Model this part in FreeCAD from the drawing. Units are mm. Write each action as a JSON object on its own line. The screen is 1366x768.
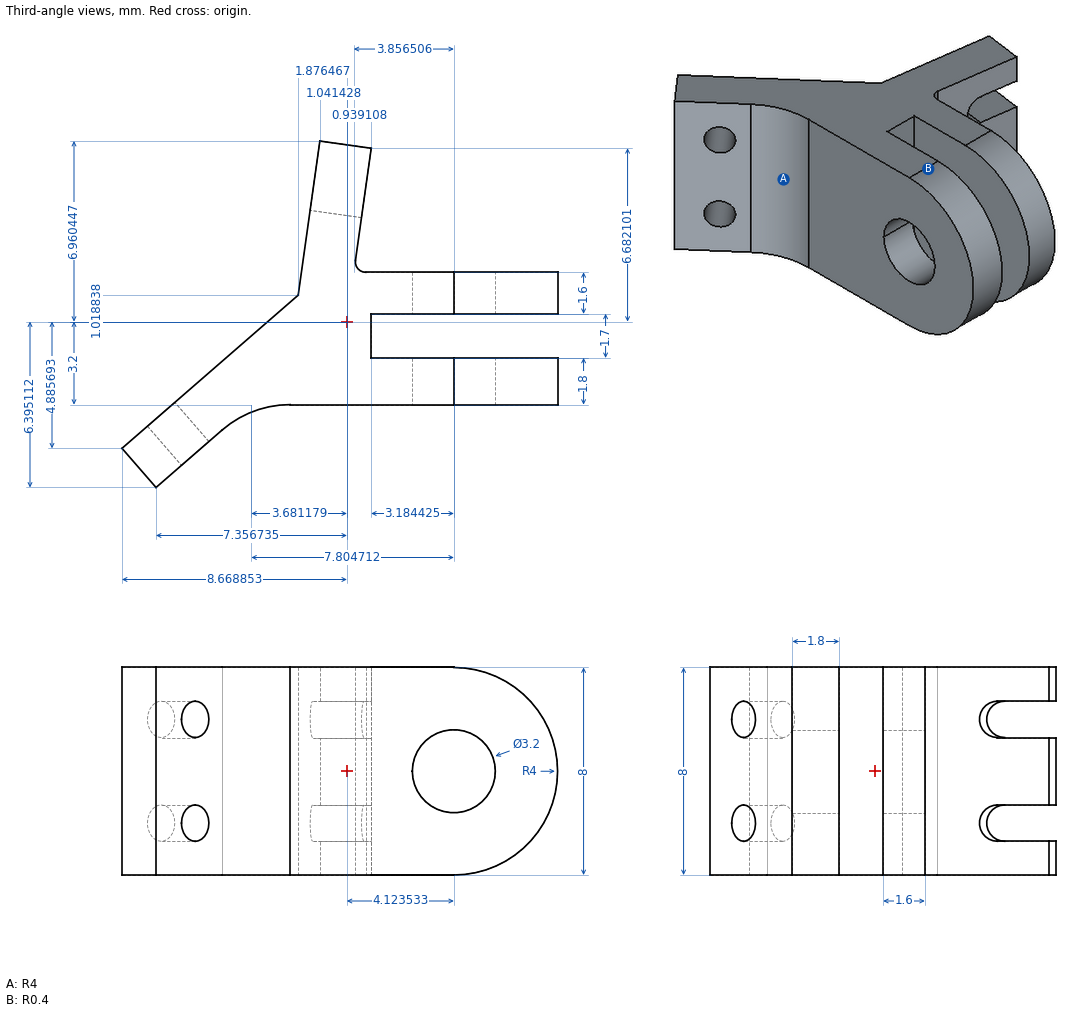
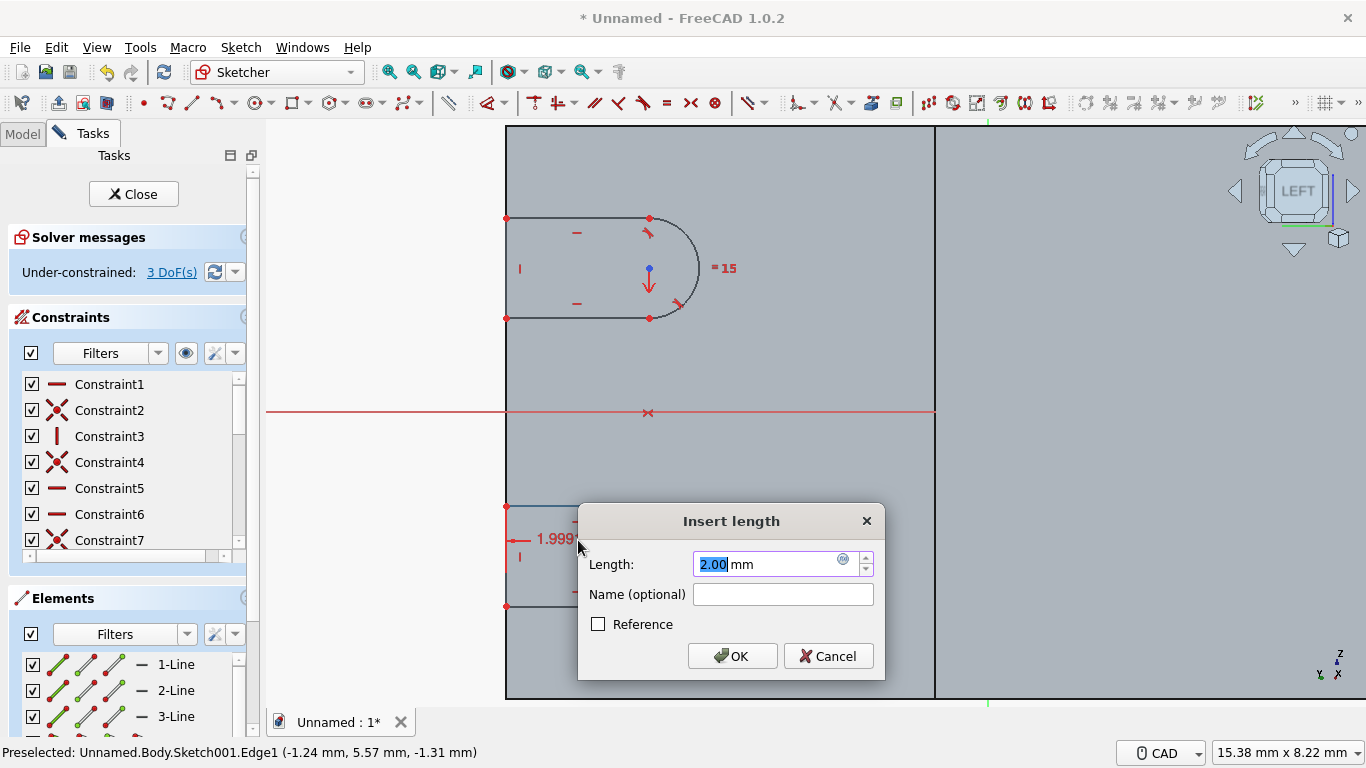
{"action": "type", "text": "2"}
{"action": "key", "text": "Return"}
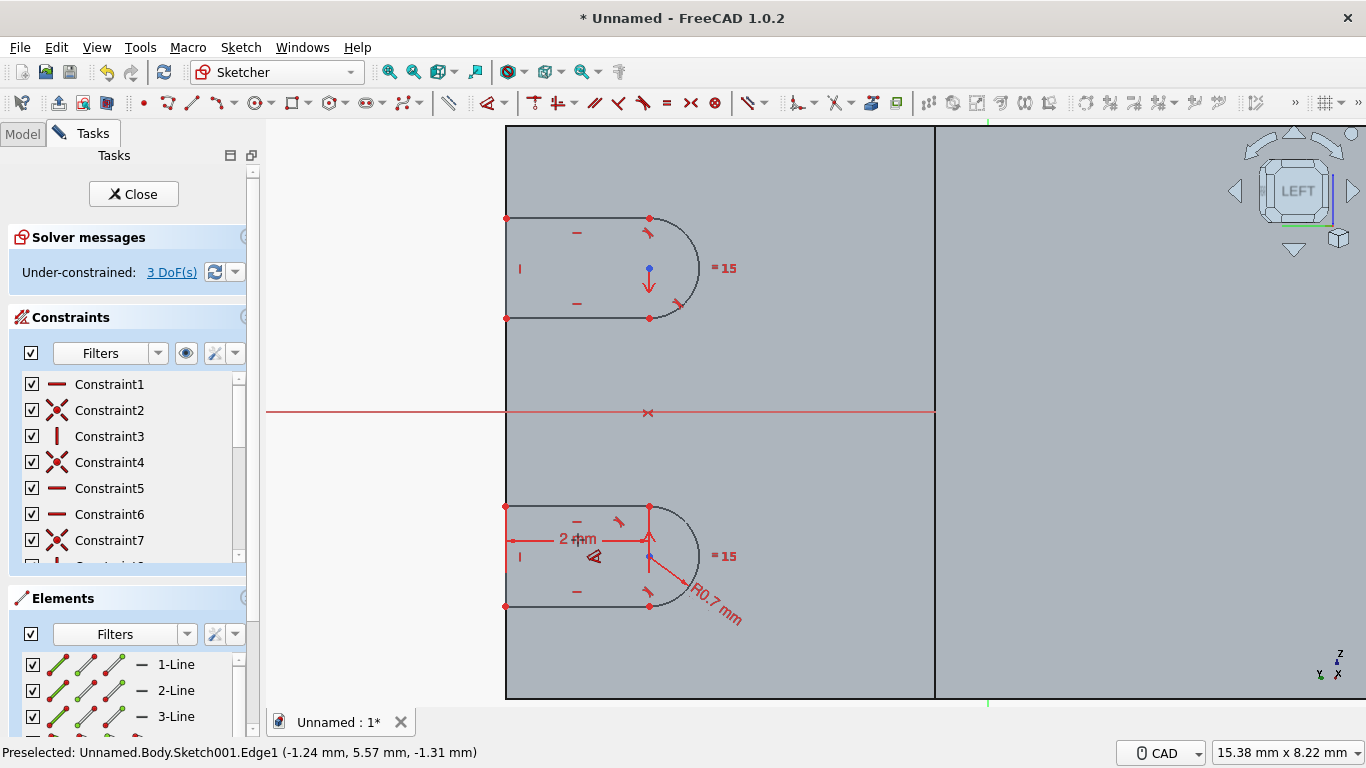
{"action": "left_click", "coordinate": [606, 218]}
{"action": "left_click", "coordinate": [578, 184]}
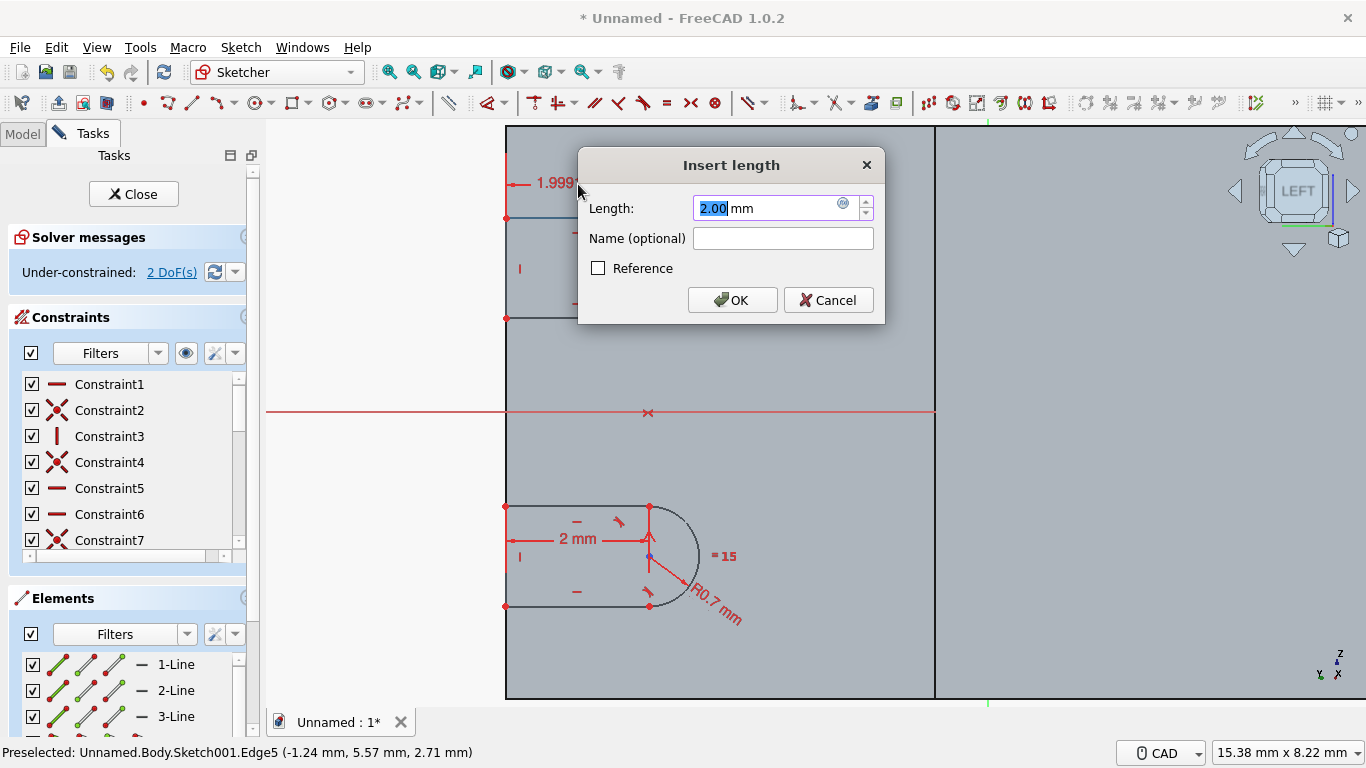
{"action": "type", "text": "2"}
{"action": "key", "text": "Return"}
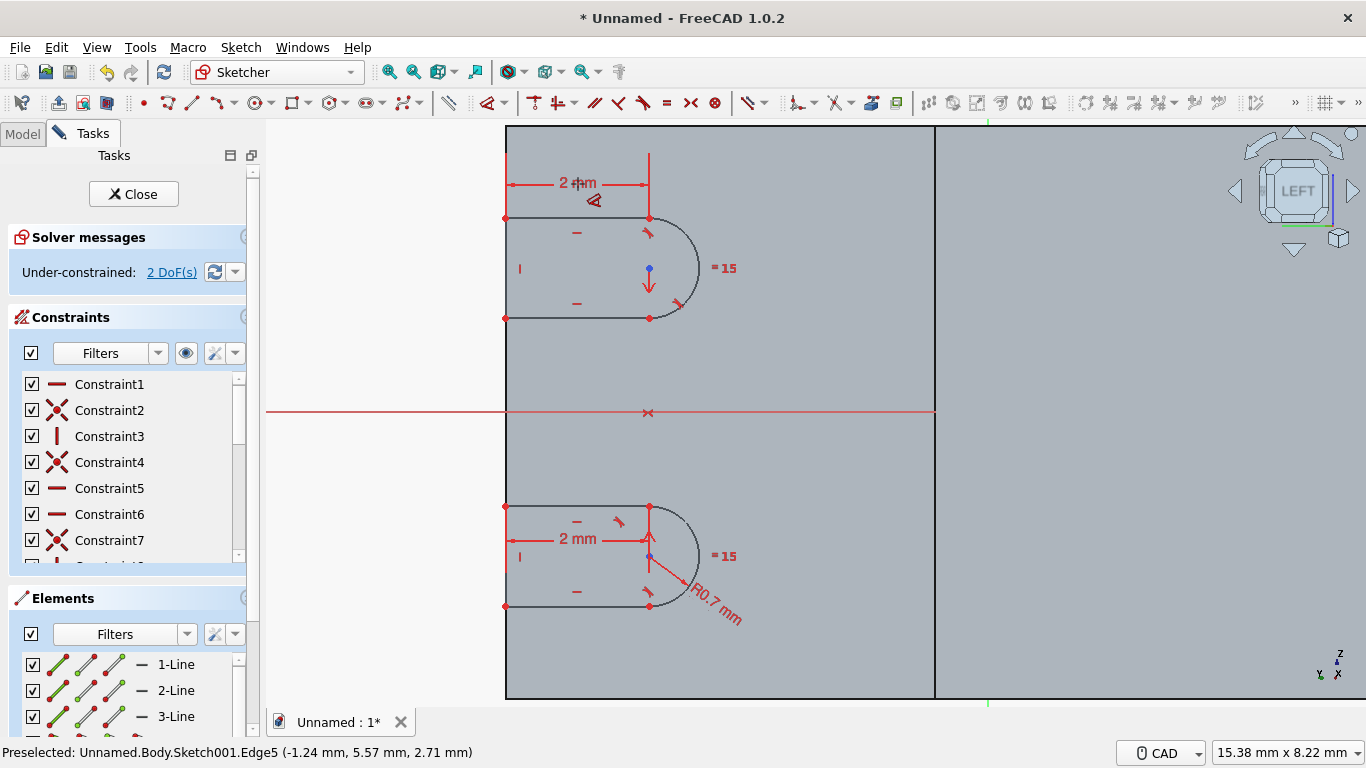
{"action": "left_click", "coordinate": [649, 557]}
{"action": "left_click", "coordinate": [1022, 484]}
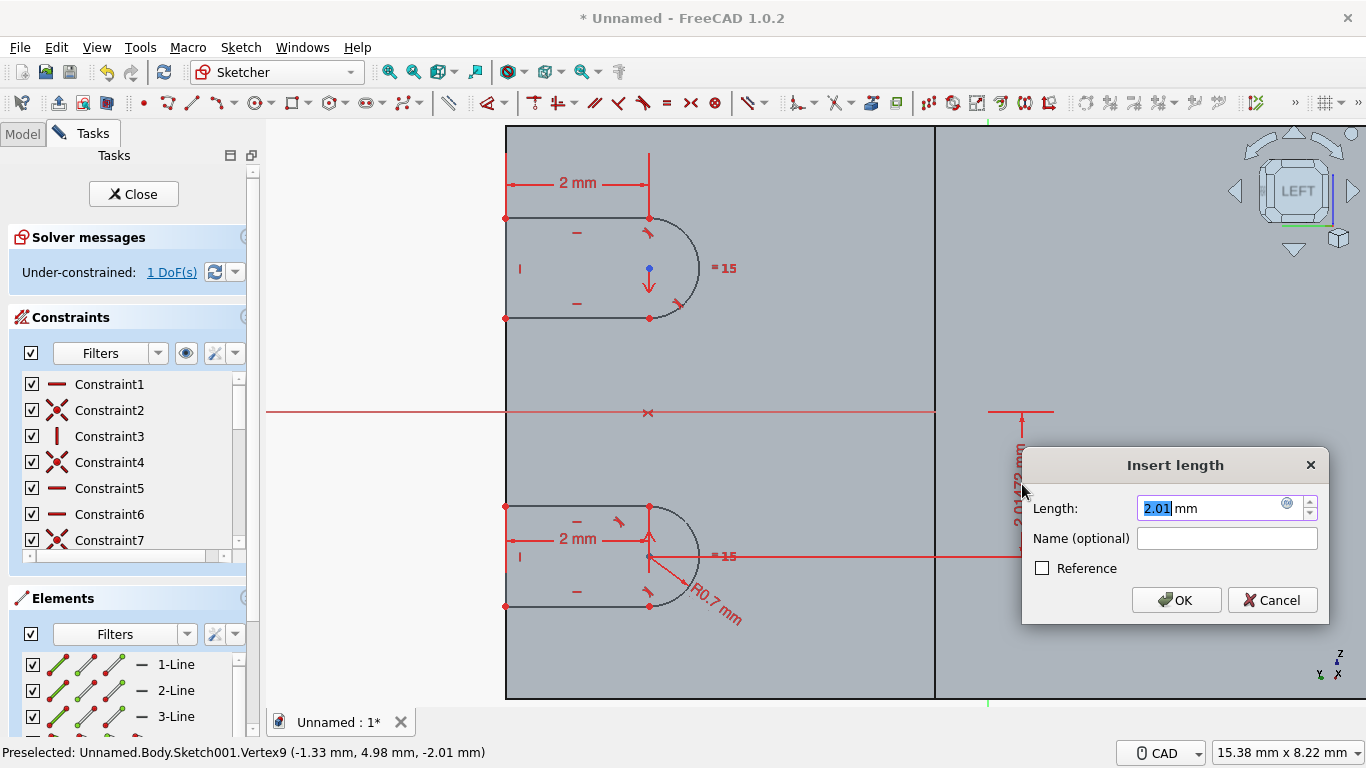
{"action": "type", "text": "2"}
{"action": "key", "text": "Return"}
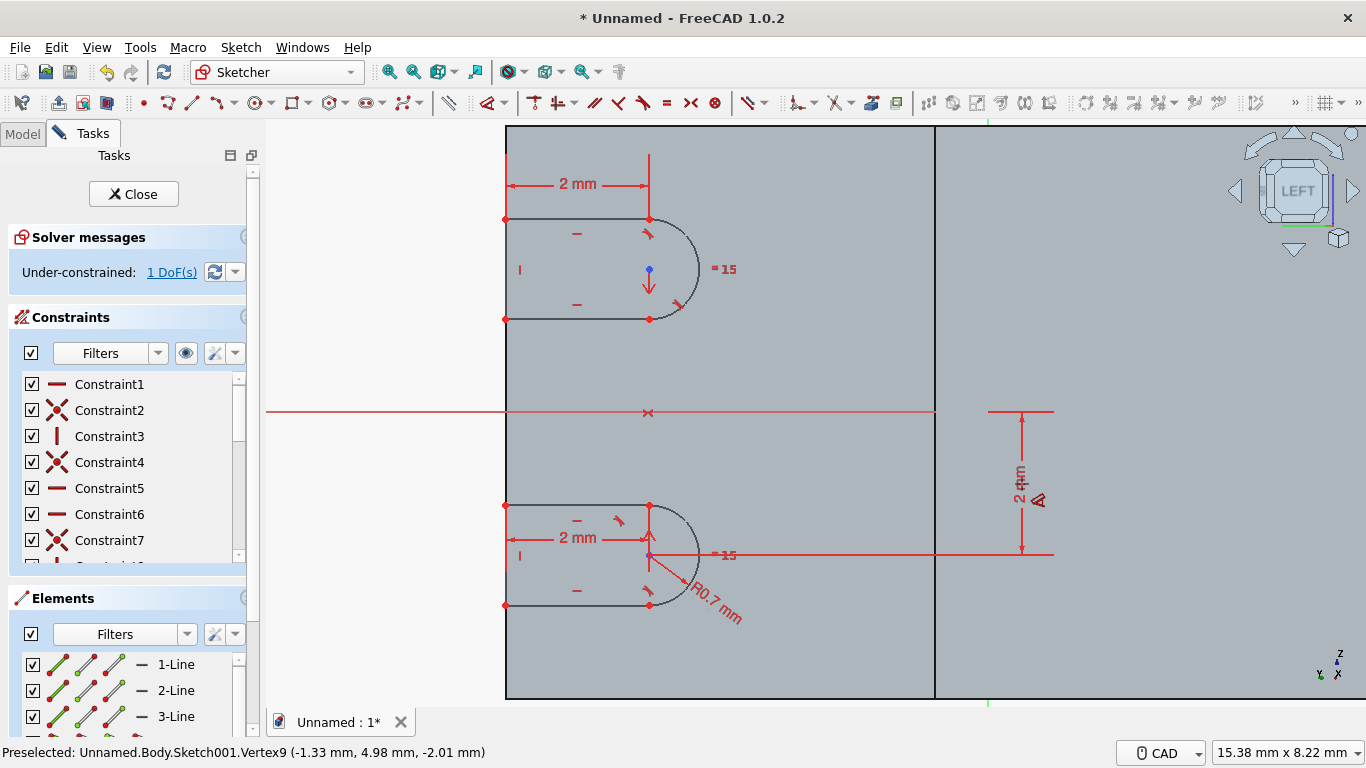
{"action": "left_click", "coordinate": [649, 505]}
{"action": "left_click", "coordinate": [819, 539]}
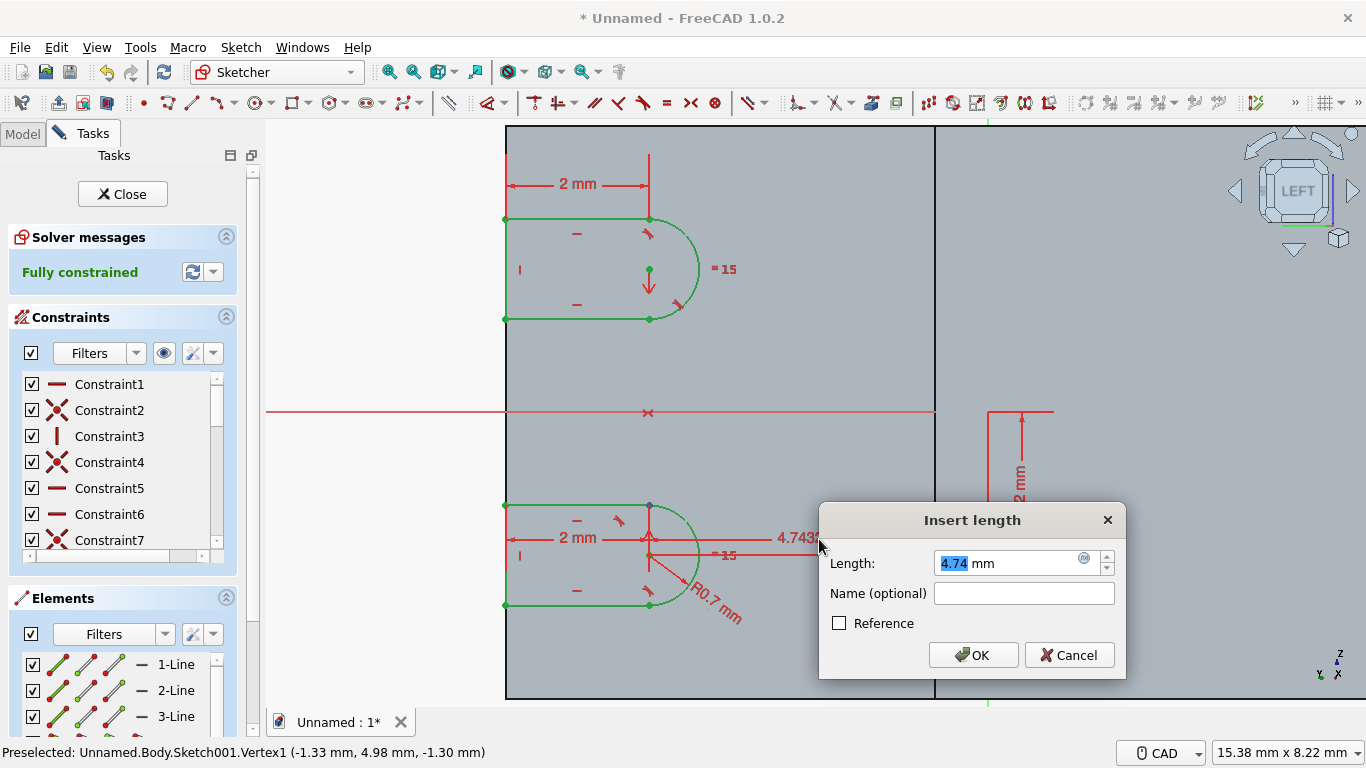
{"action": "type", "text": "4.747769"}
{"action": "key", "text": "Return"}
{"action": "key", "text": "Escape"}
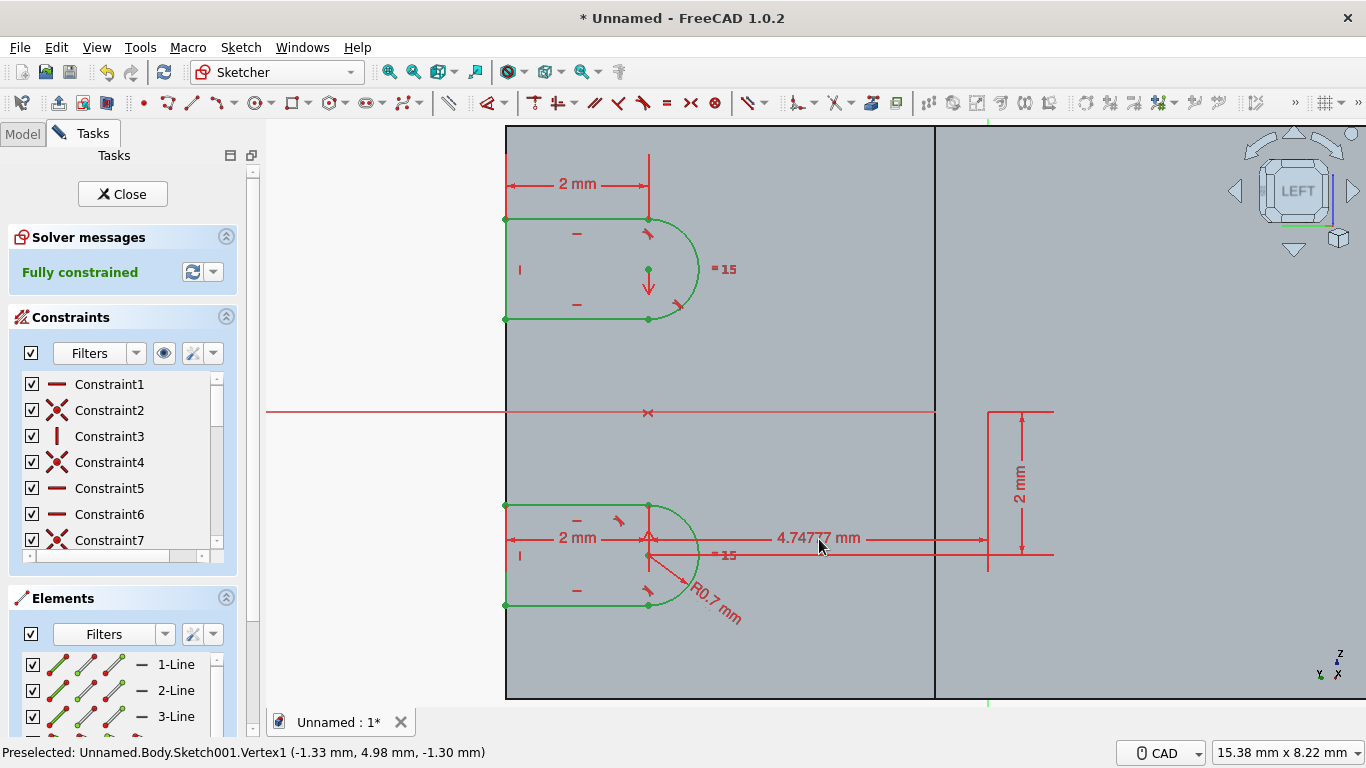
{"action": "left_click", "coordinate": [123, 194]}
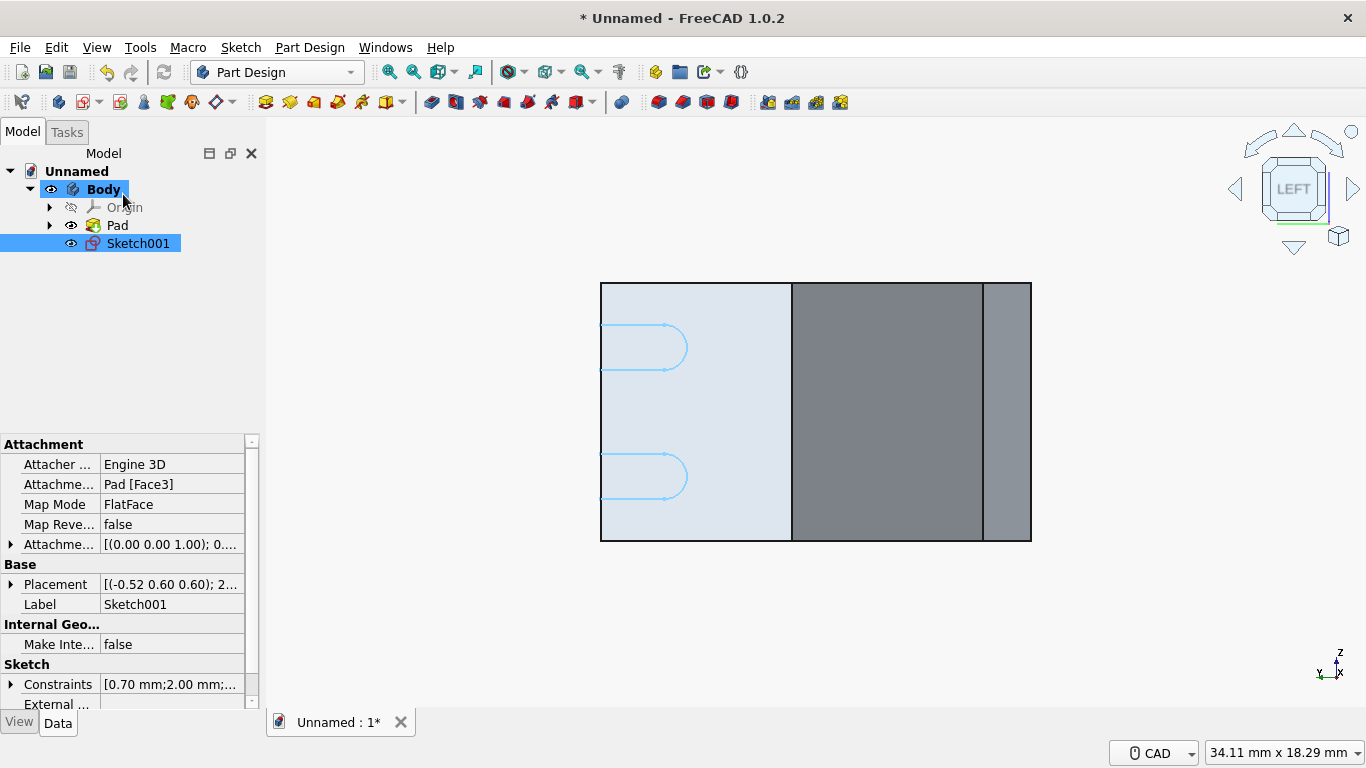
{"action": "left_click", "coordinate": [432, 102]}